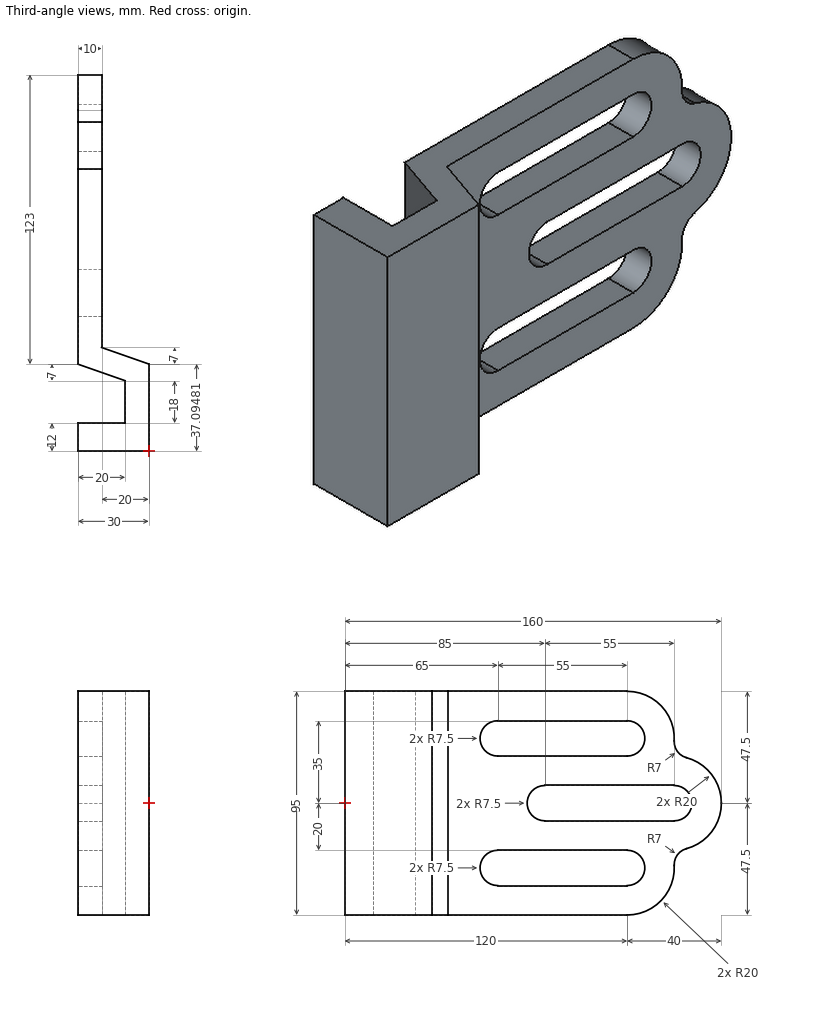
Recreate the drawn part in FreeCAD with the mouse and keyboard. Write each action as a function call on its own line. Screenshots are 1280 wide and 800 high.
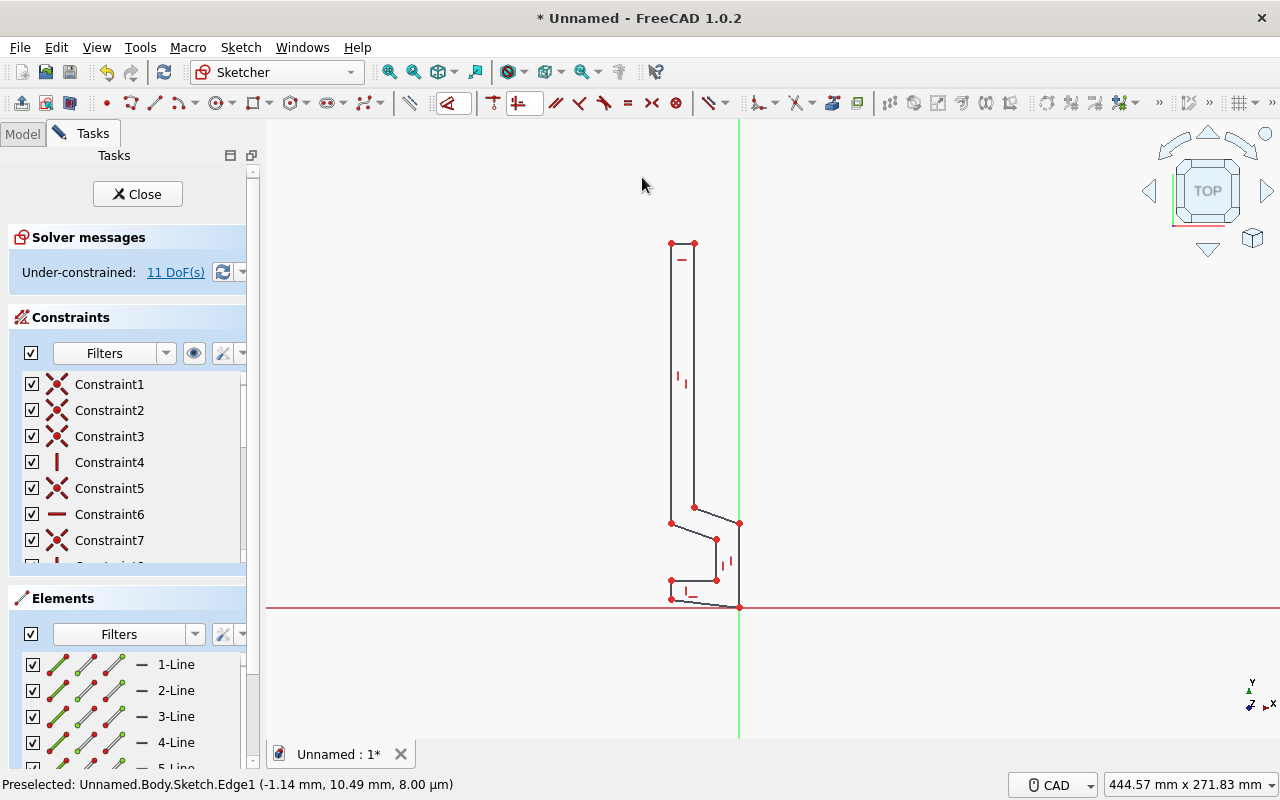
click(719, 606)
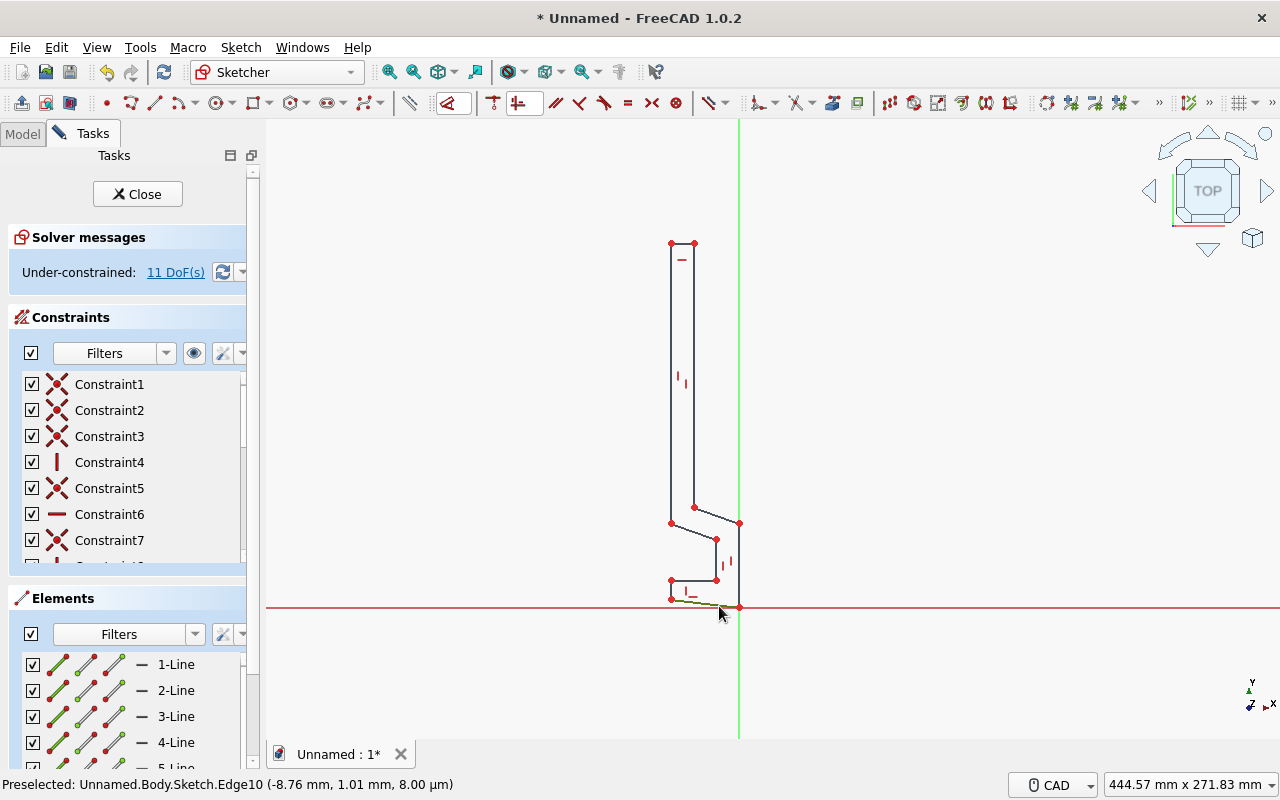
click(538, 104)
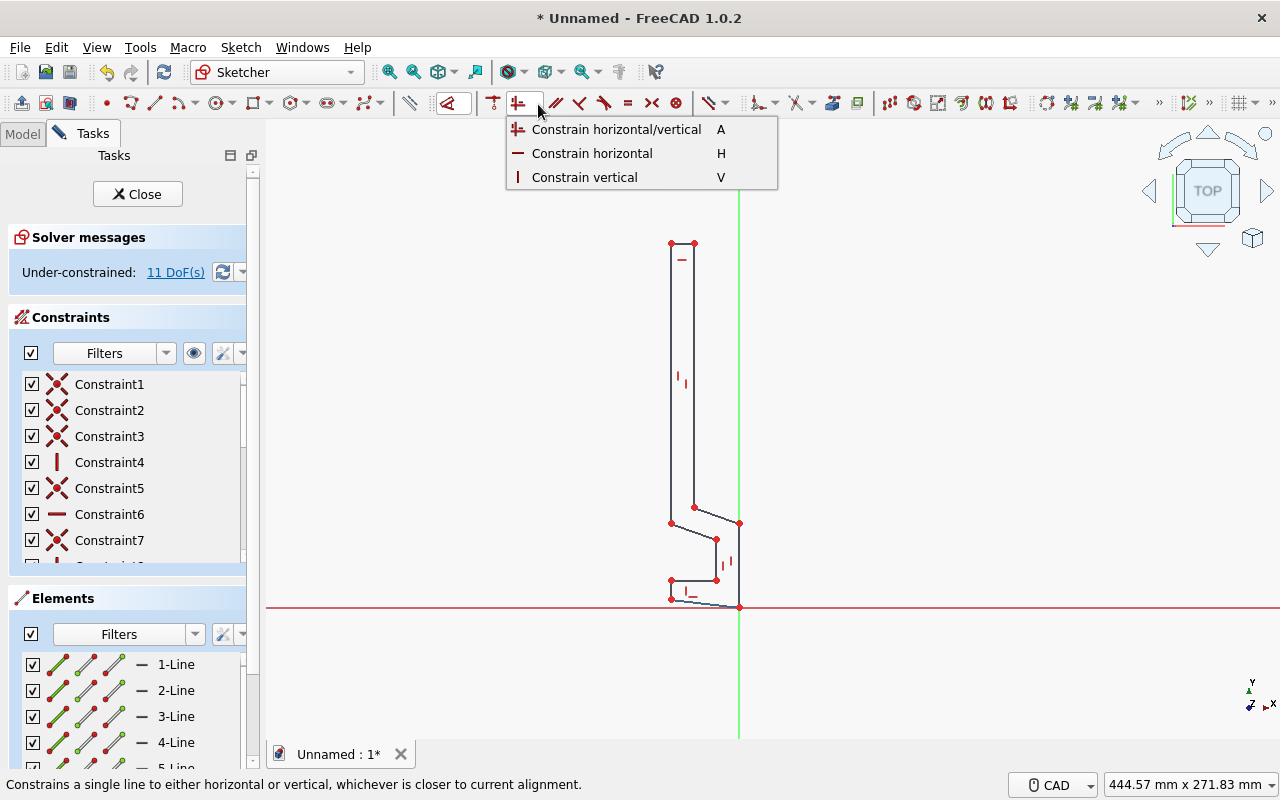
click(642, 153)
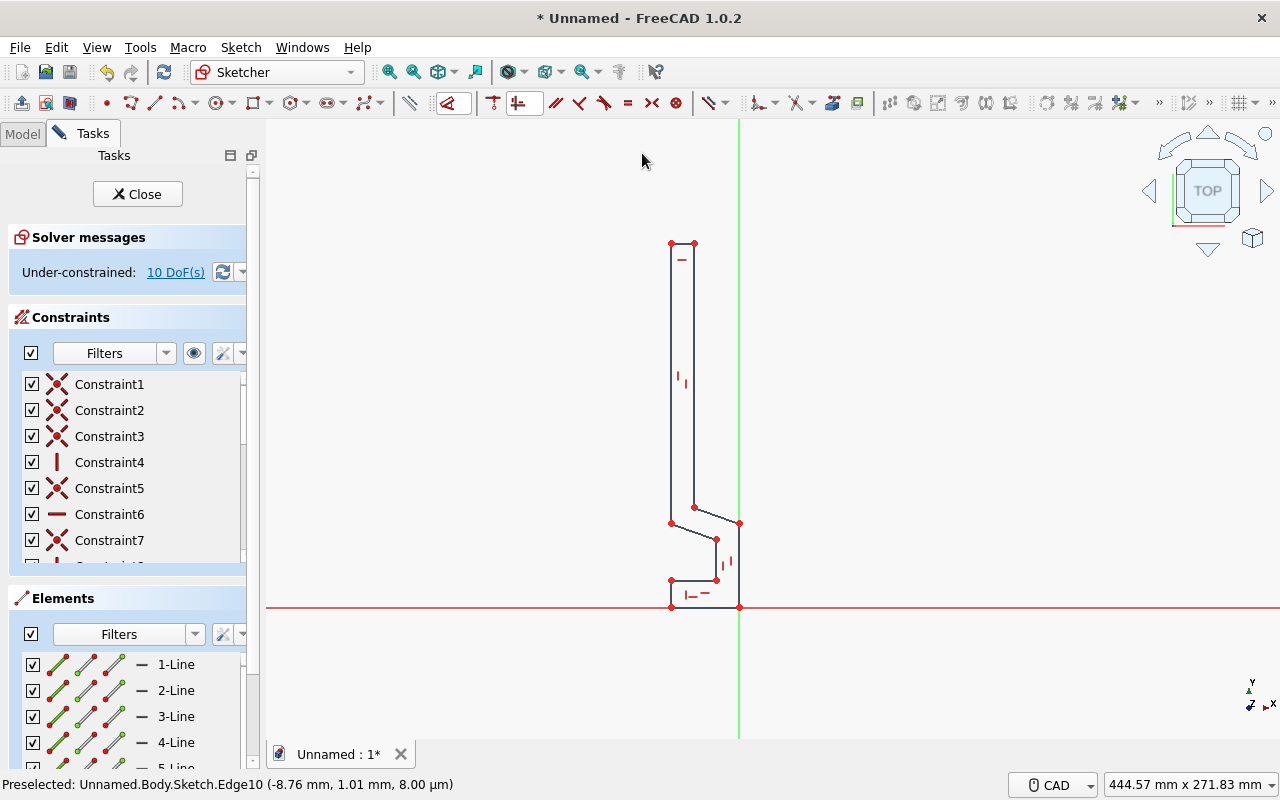
key(d)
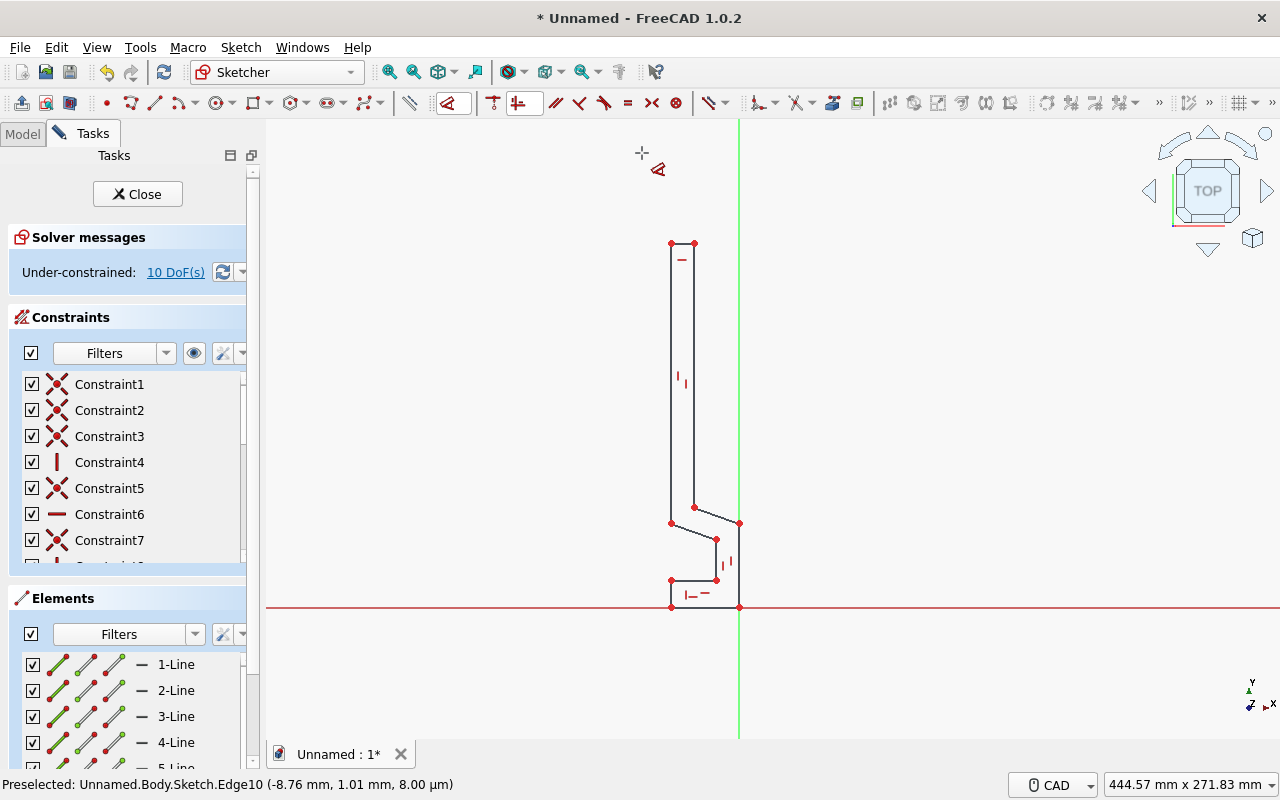
scroll(685, 244, up, 3)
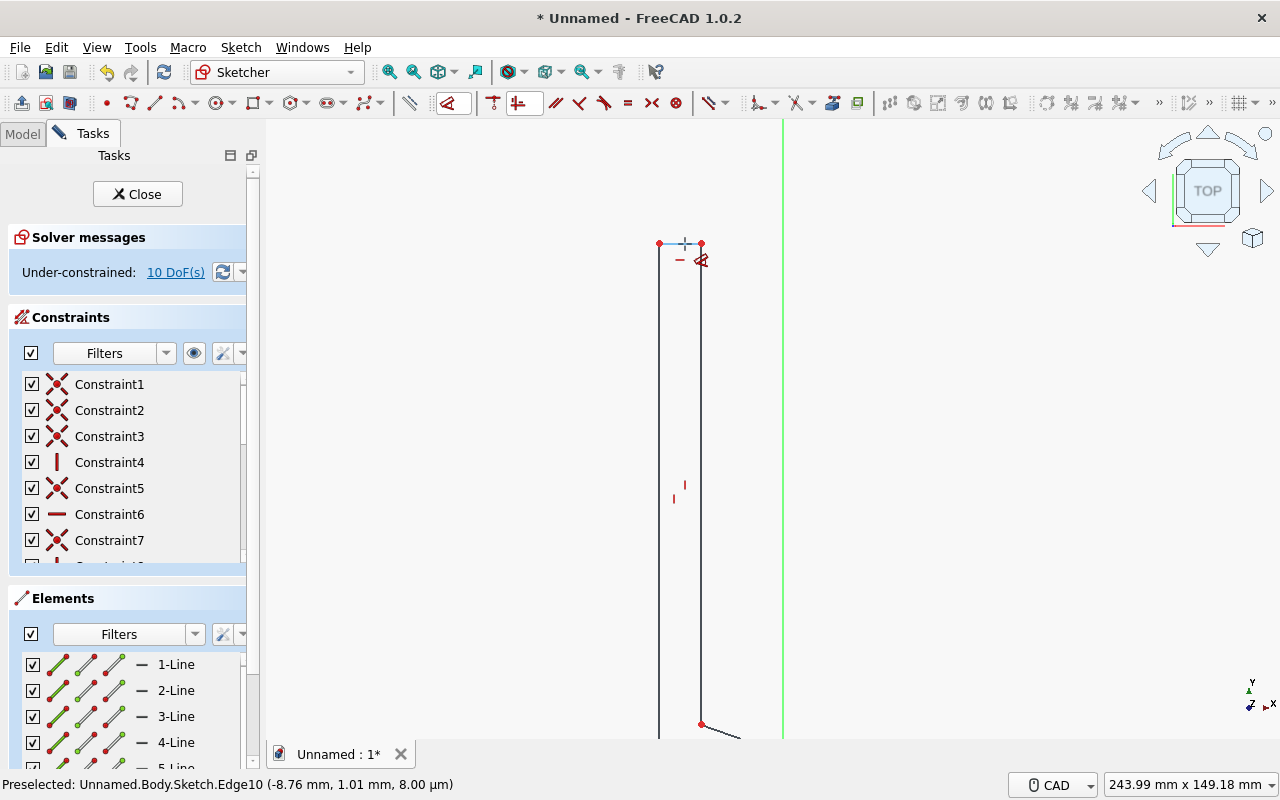
click(684, 244)
click(680, 210)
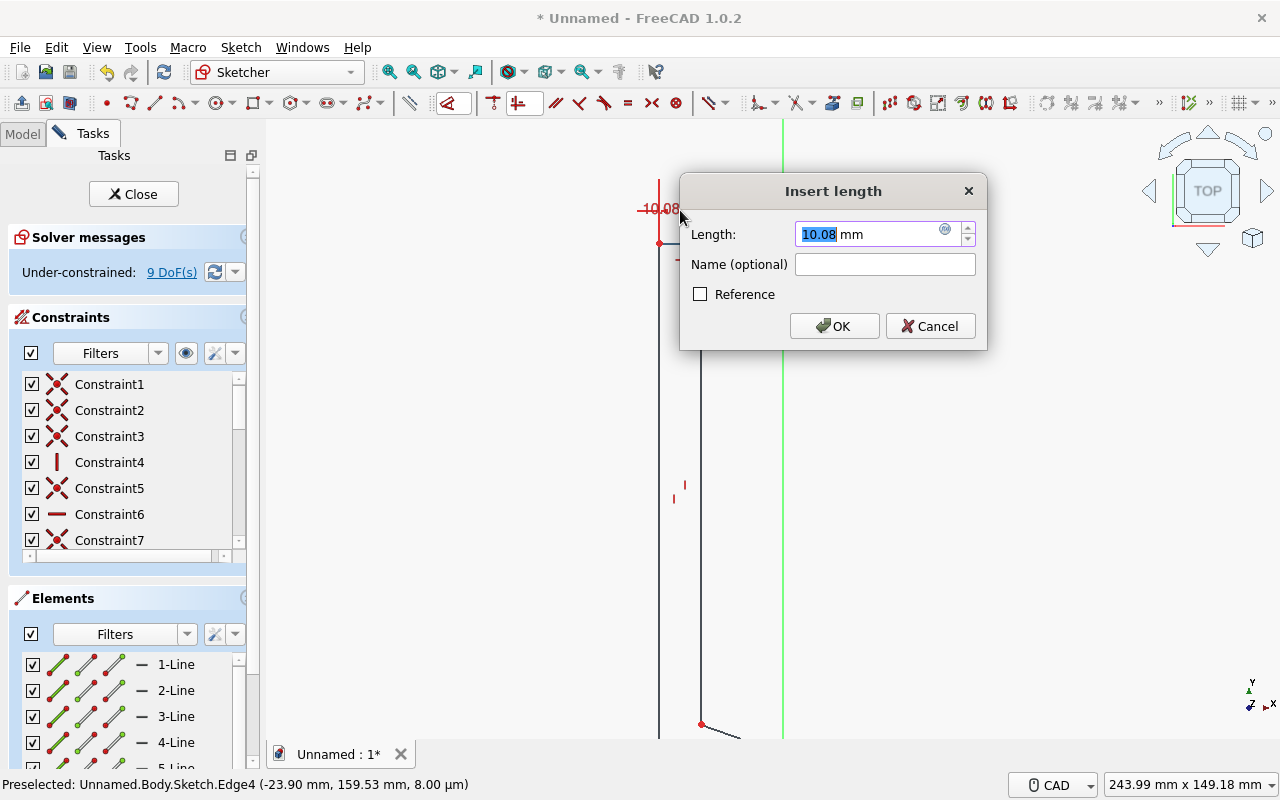
text(10)
key(Return)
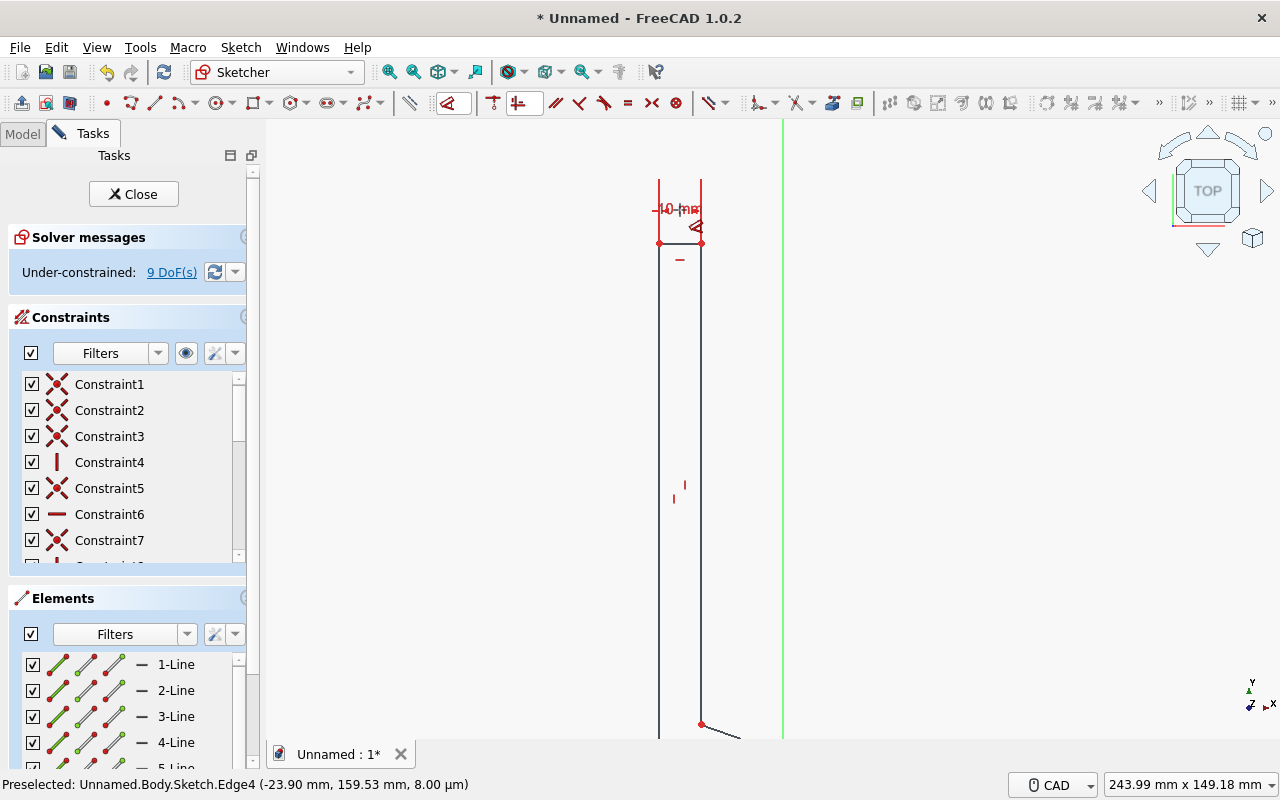
scroll(684, 252, down, 3)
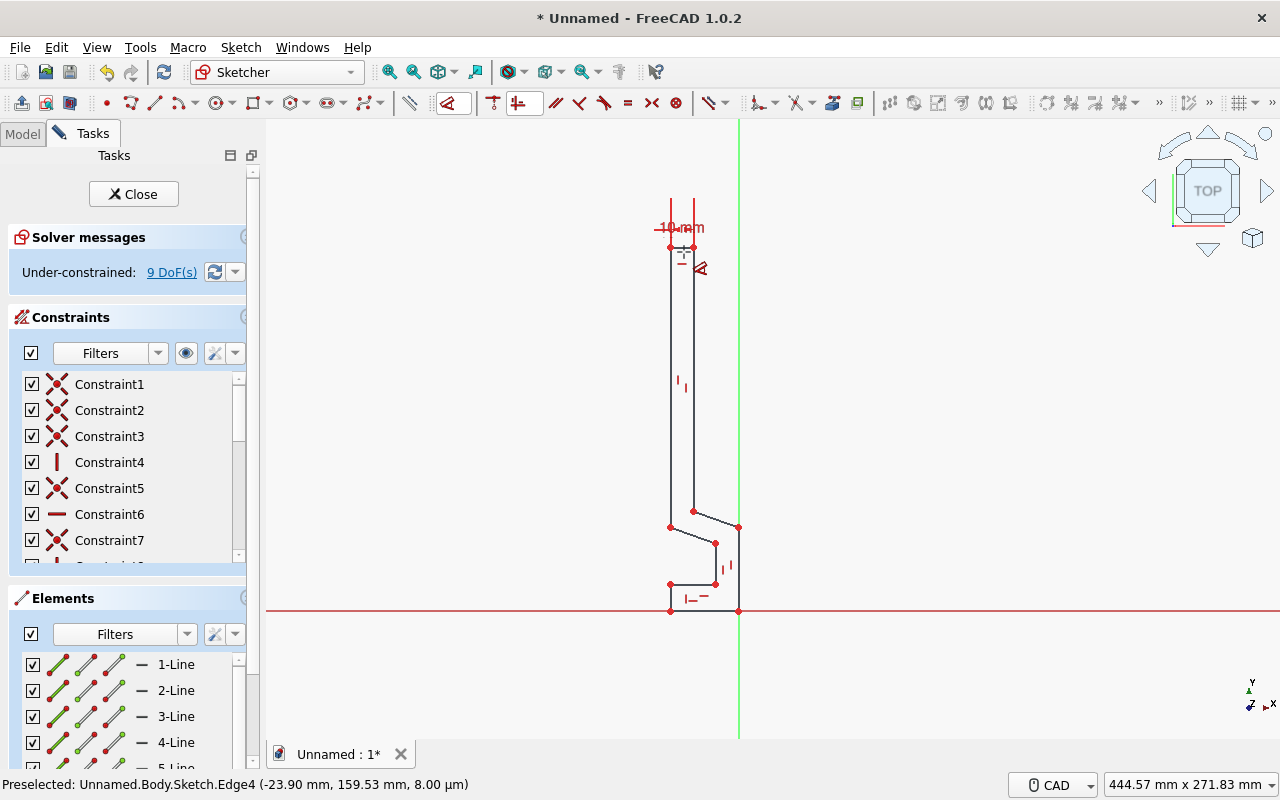
click(716, 556)
click(682, 564)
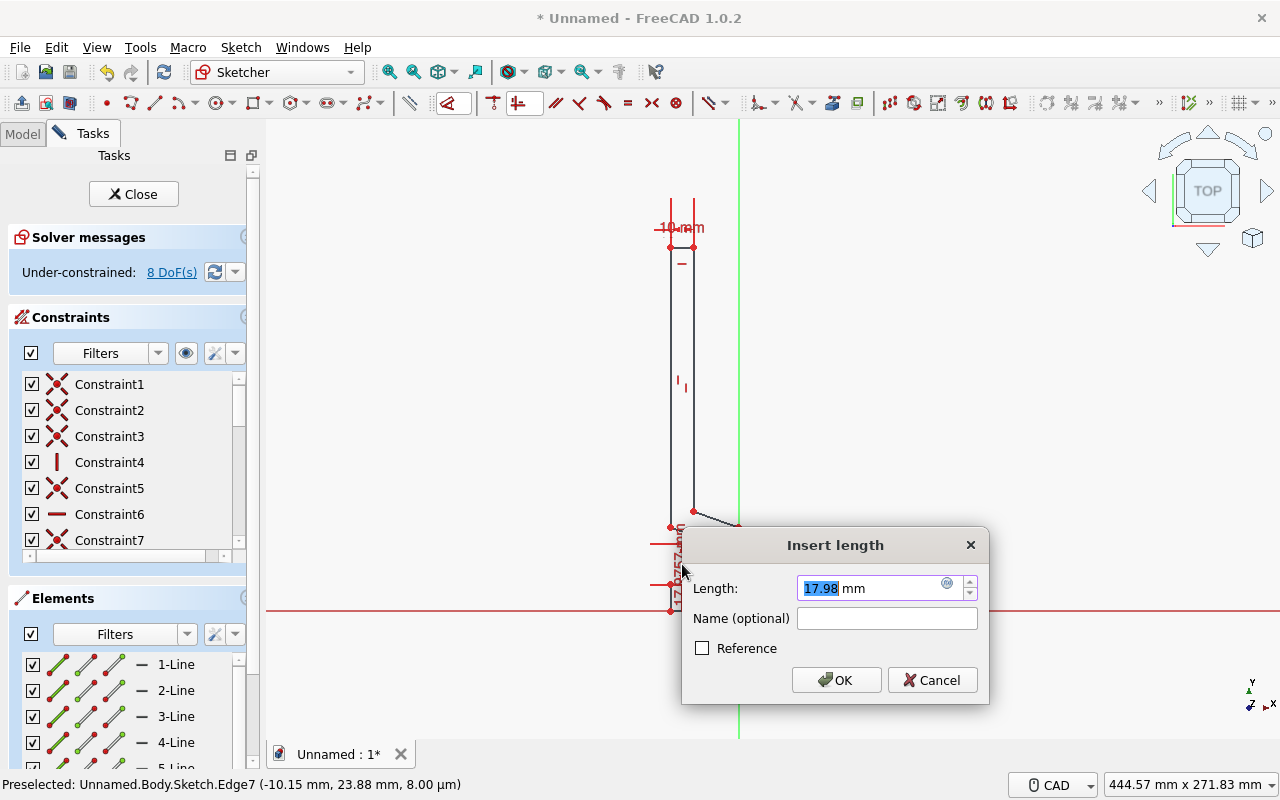
text(18)
key(Return)